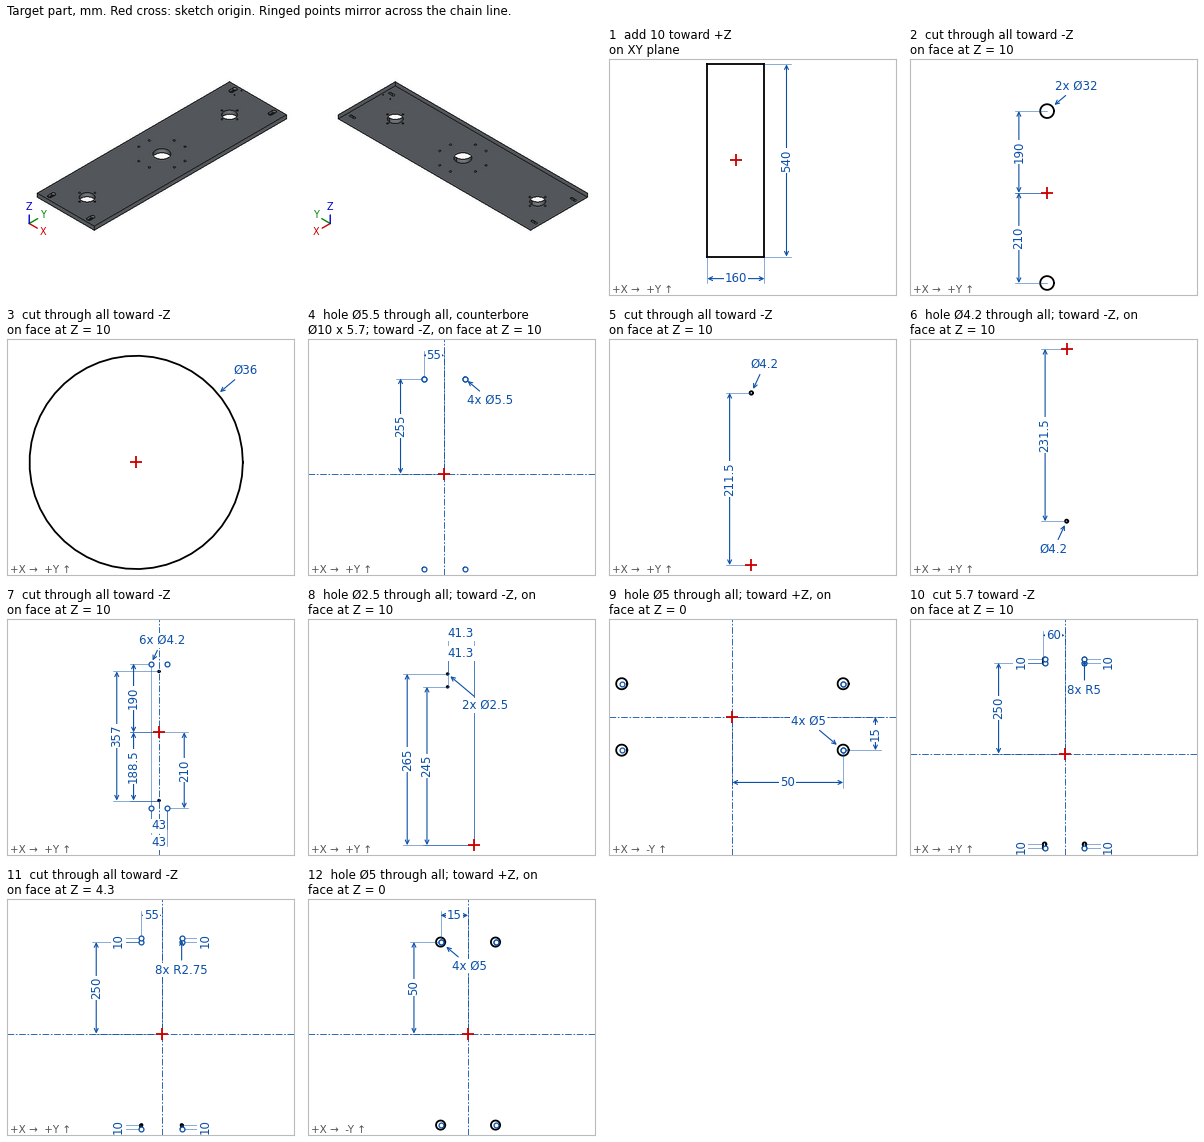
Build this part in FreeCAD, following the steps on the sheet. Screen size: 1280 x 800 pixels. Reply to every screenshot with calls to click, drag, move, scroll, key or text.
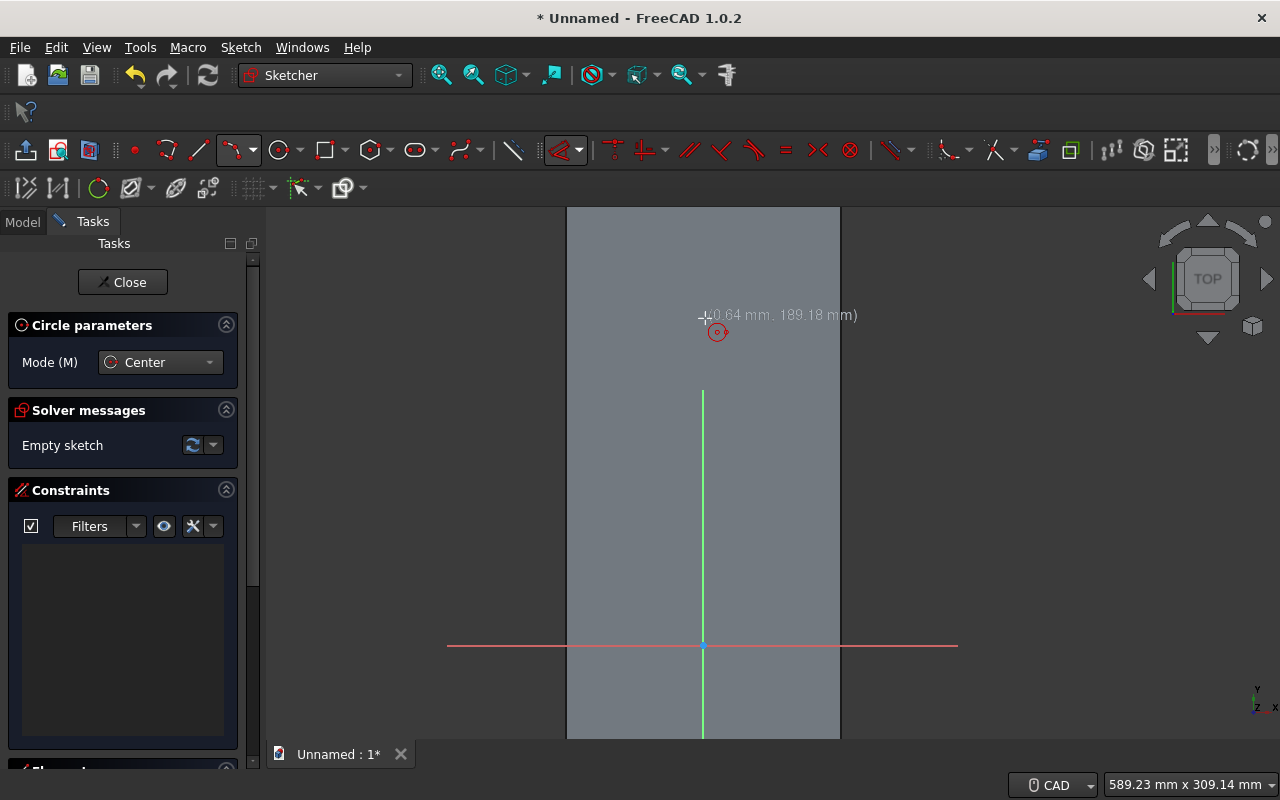
click(703, 319)
move(723, 299)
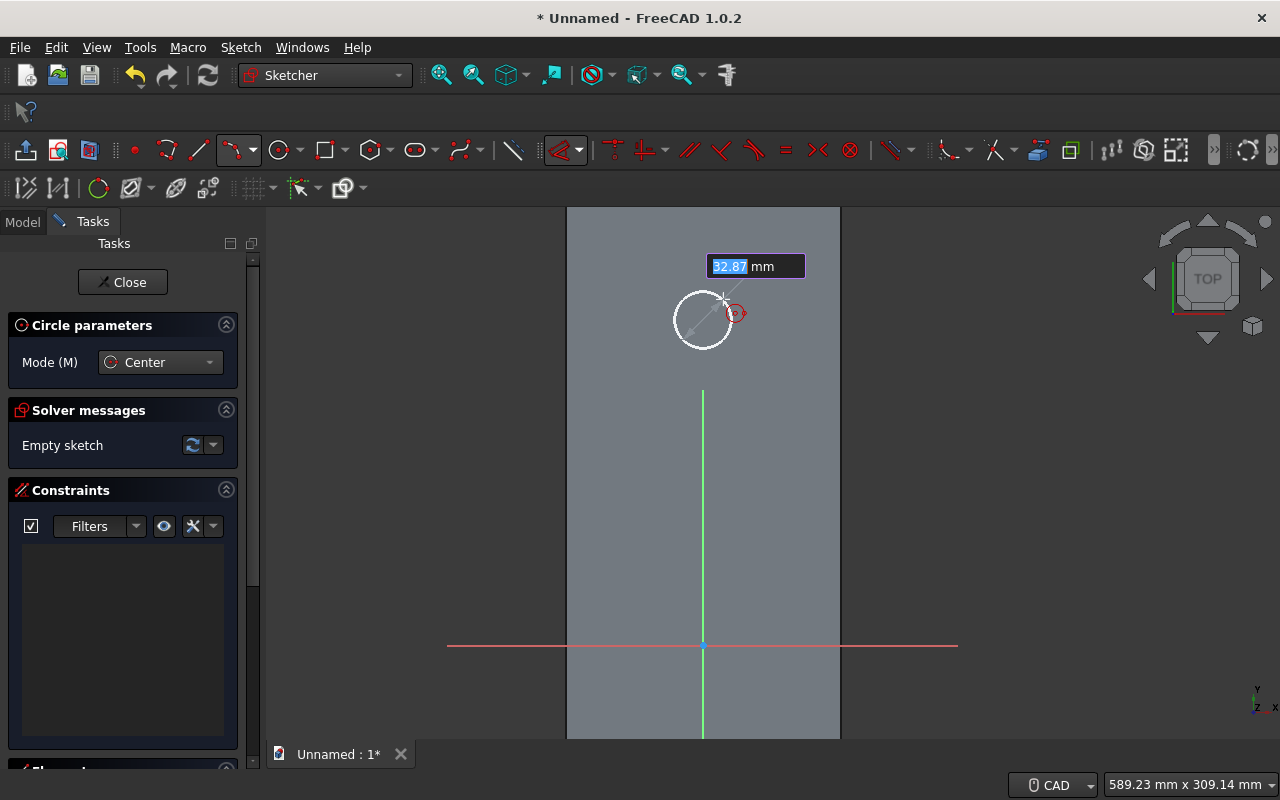
text(32)
key(Return)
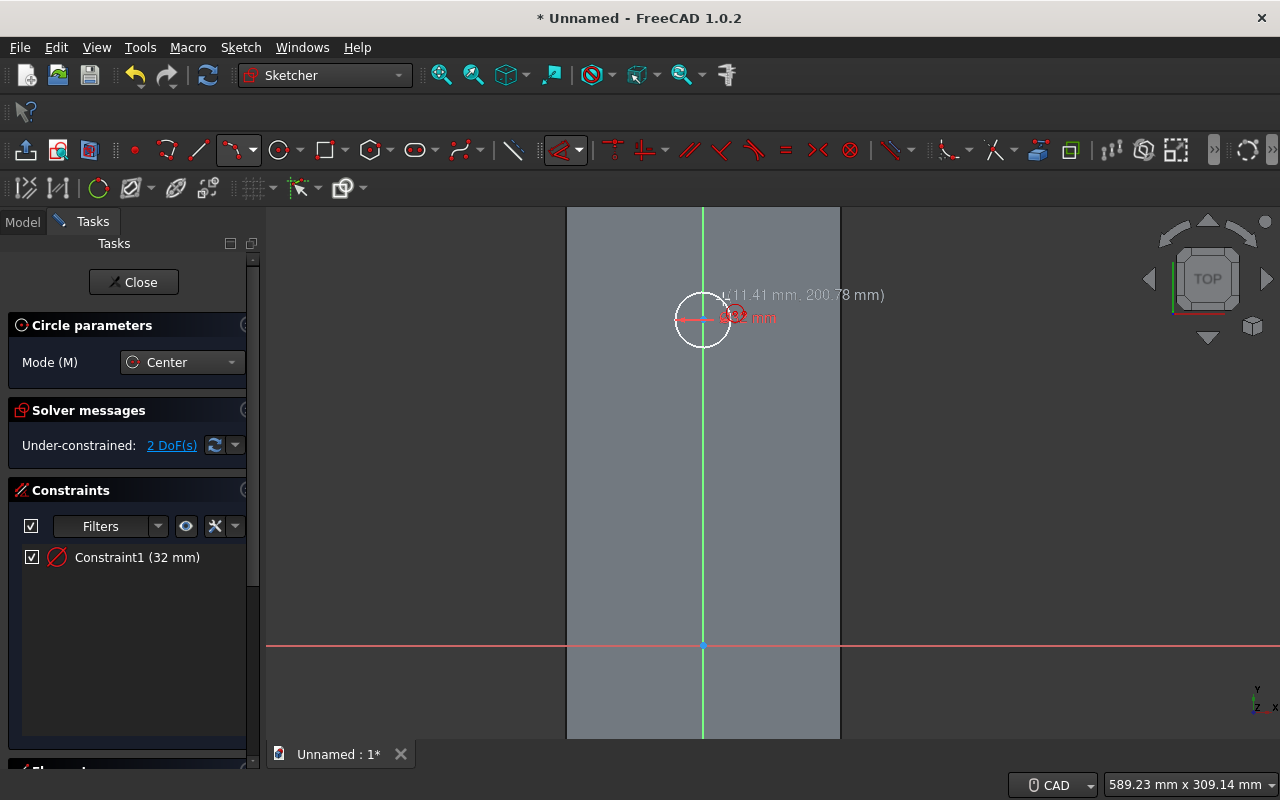
scroll(705, 318, down, 4)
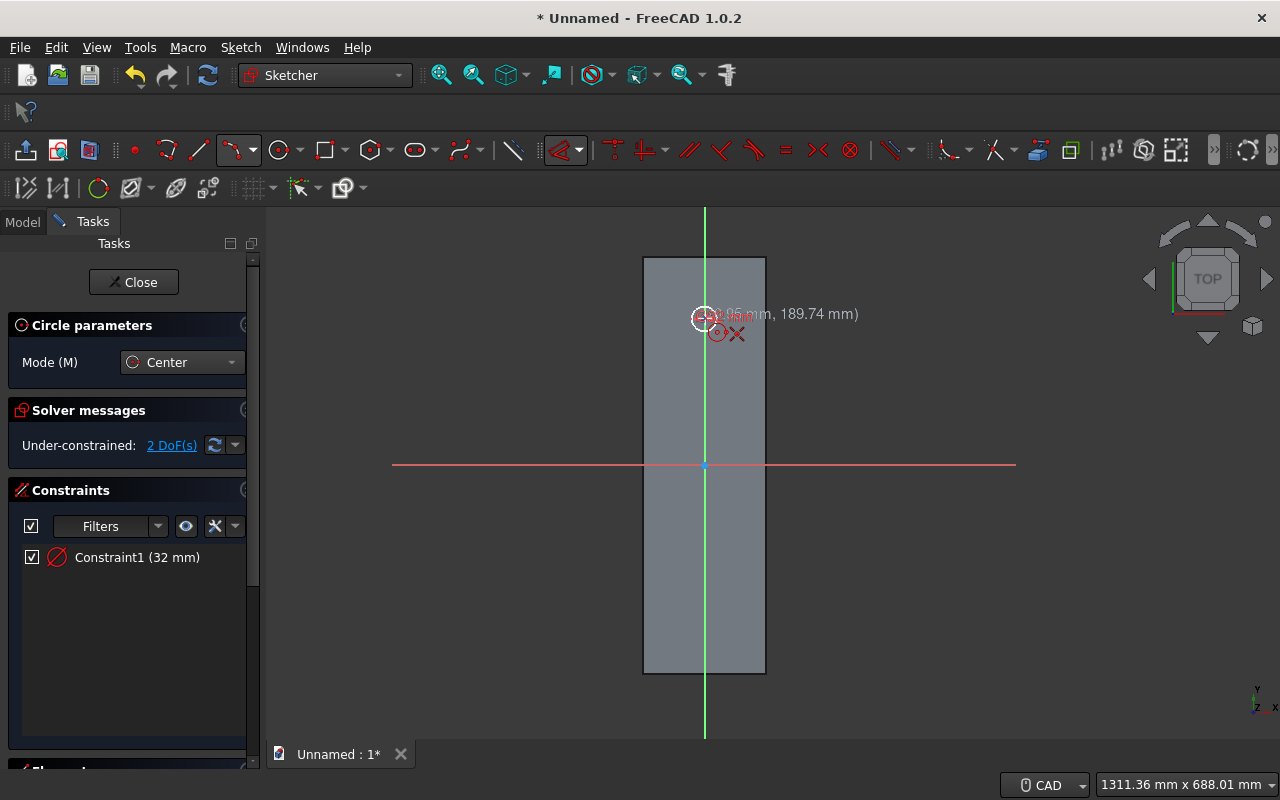
scroll(705, 628, up, 4)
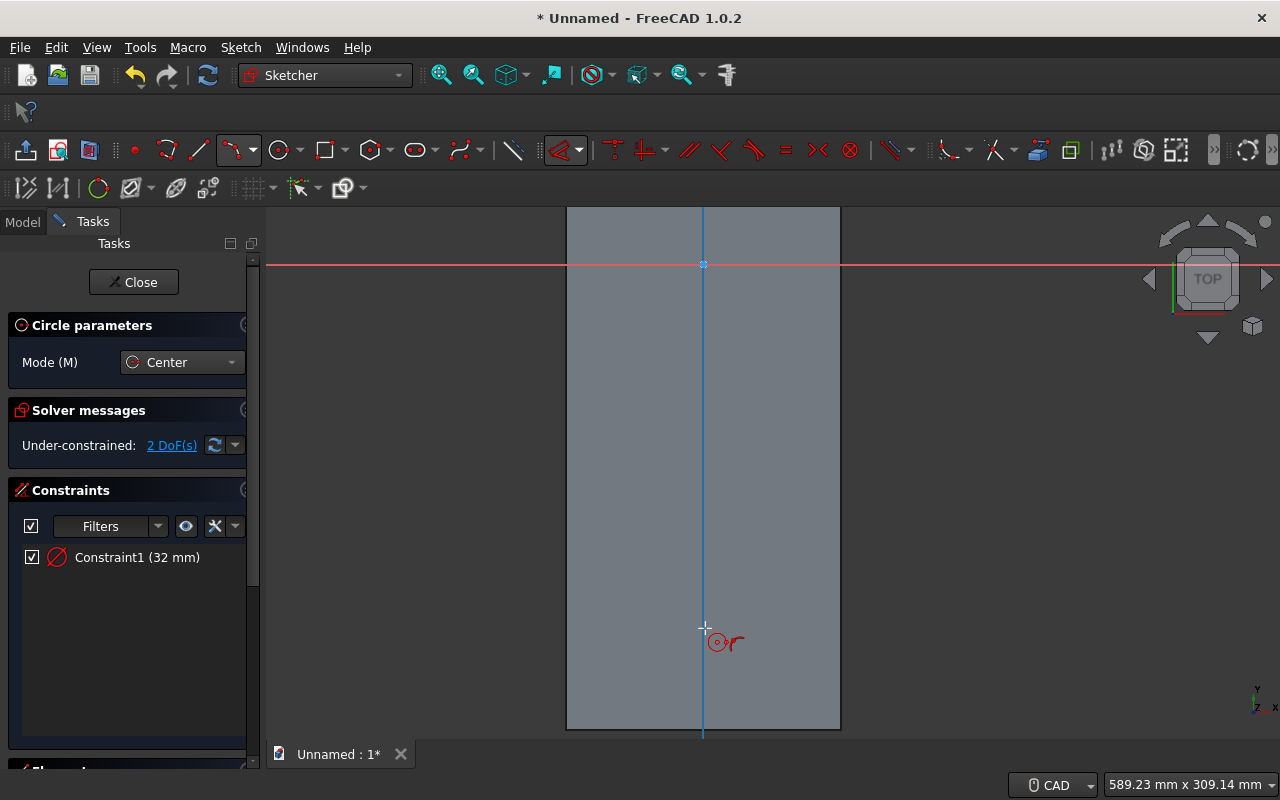
click(703, 626)
move(723, 607)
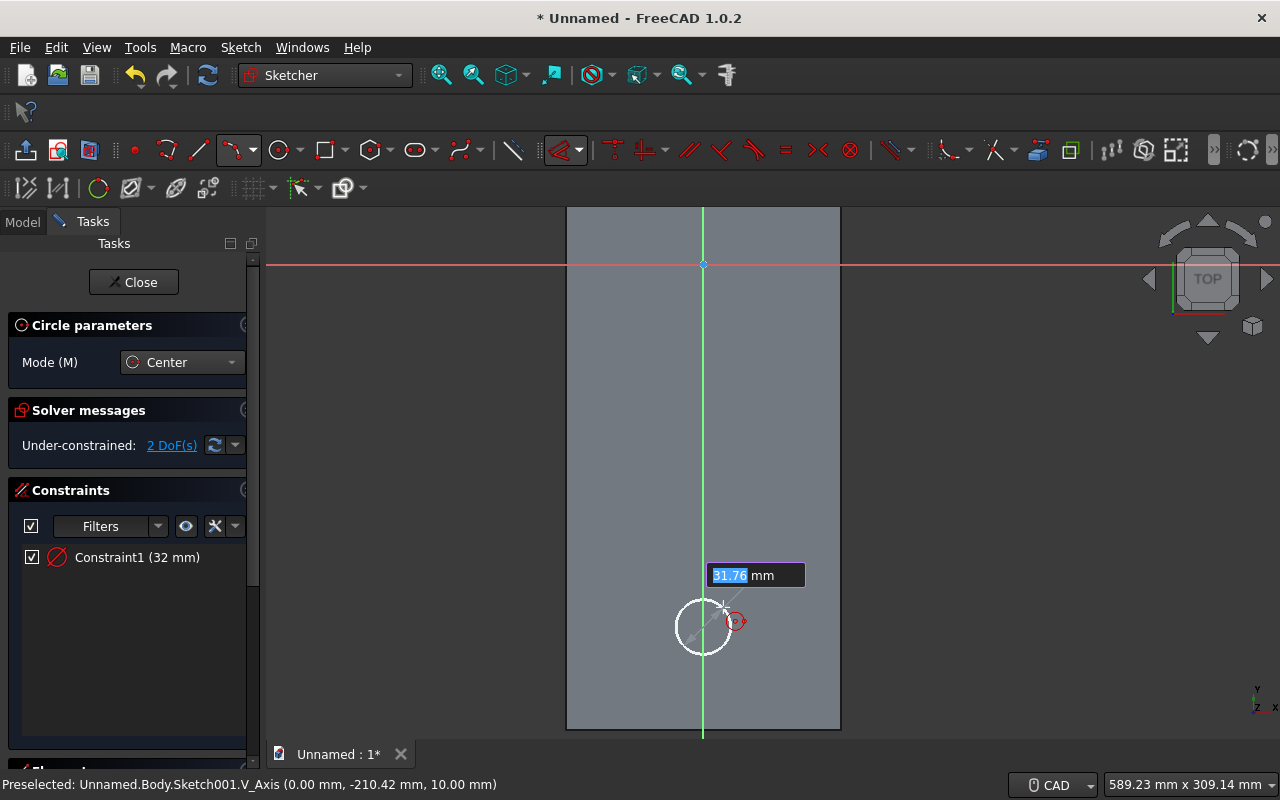
text(32)
key(Return)
key(Escape)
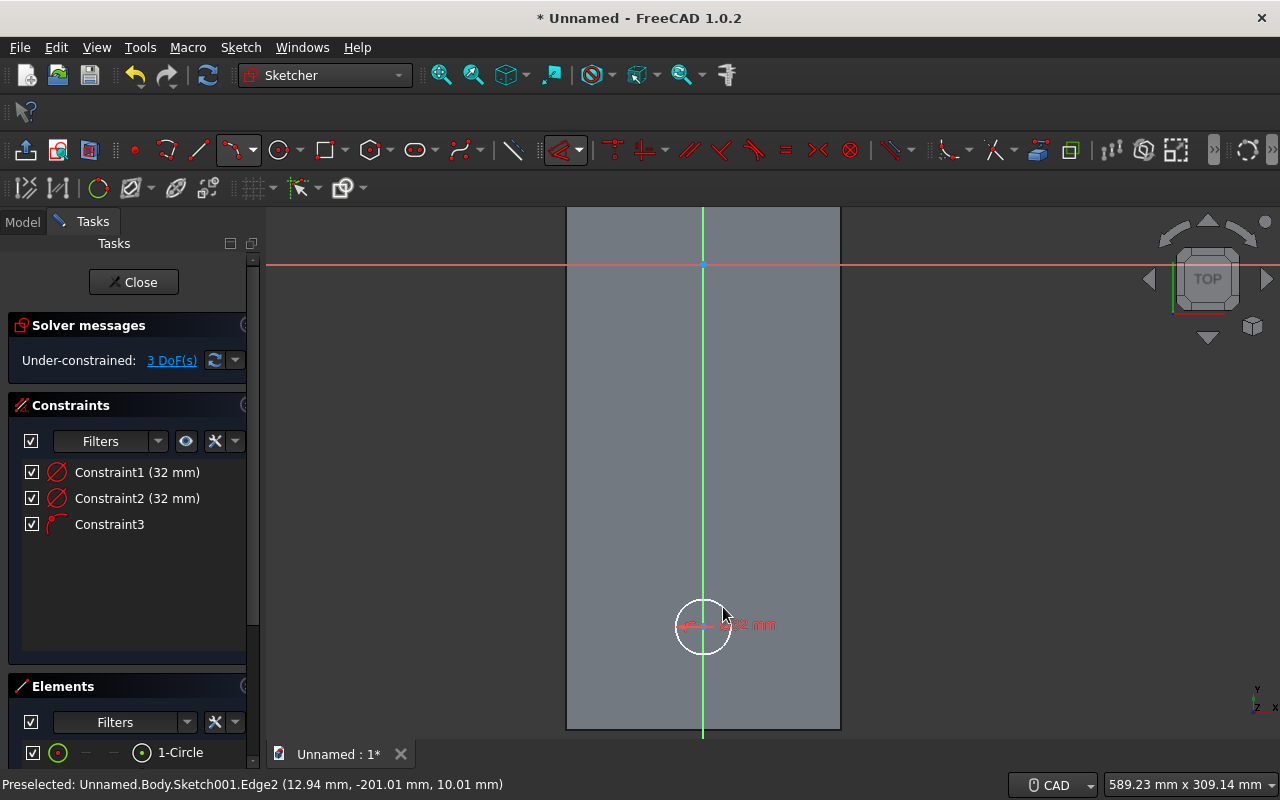
scroll(705, 629, down, 4)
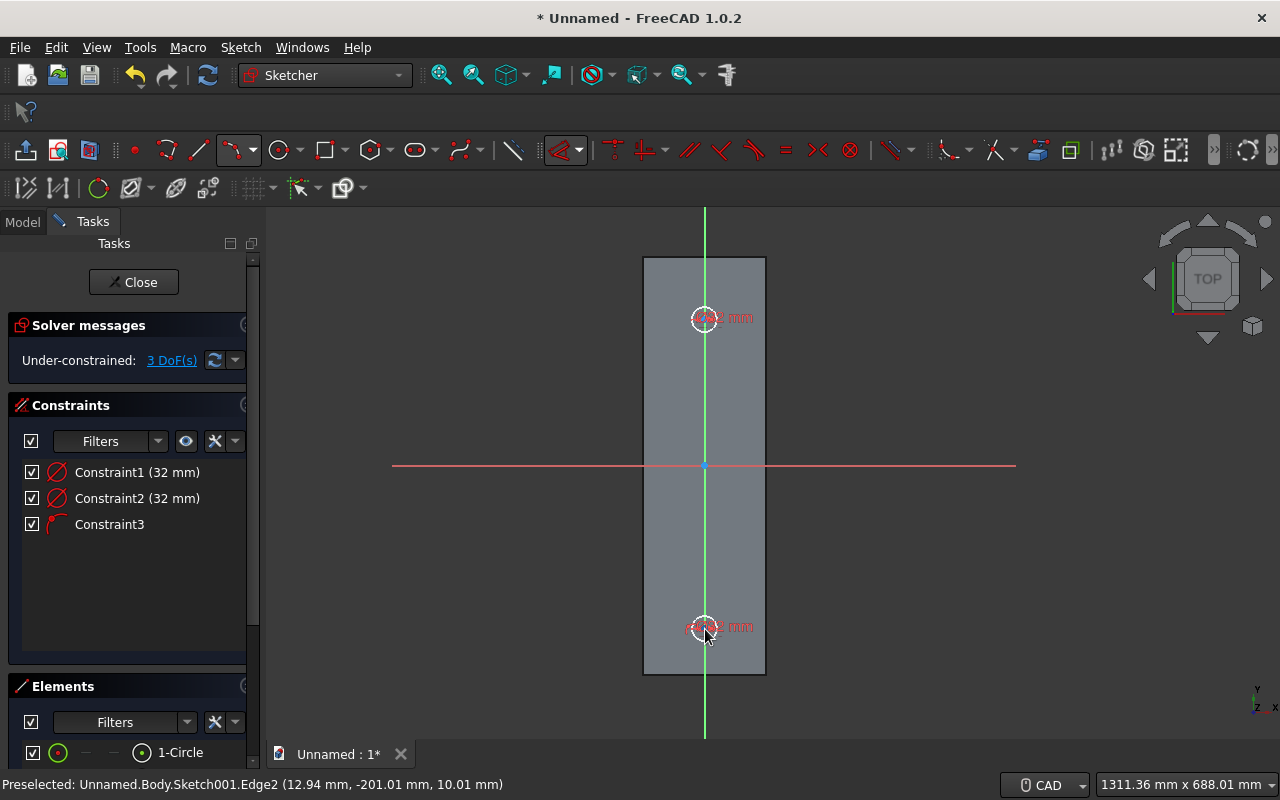
click(704, 320)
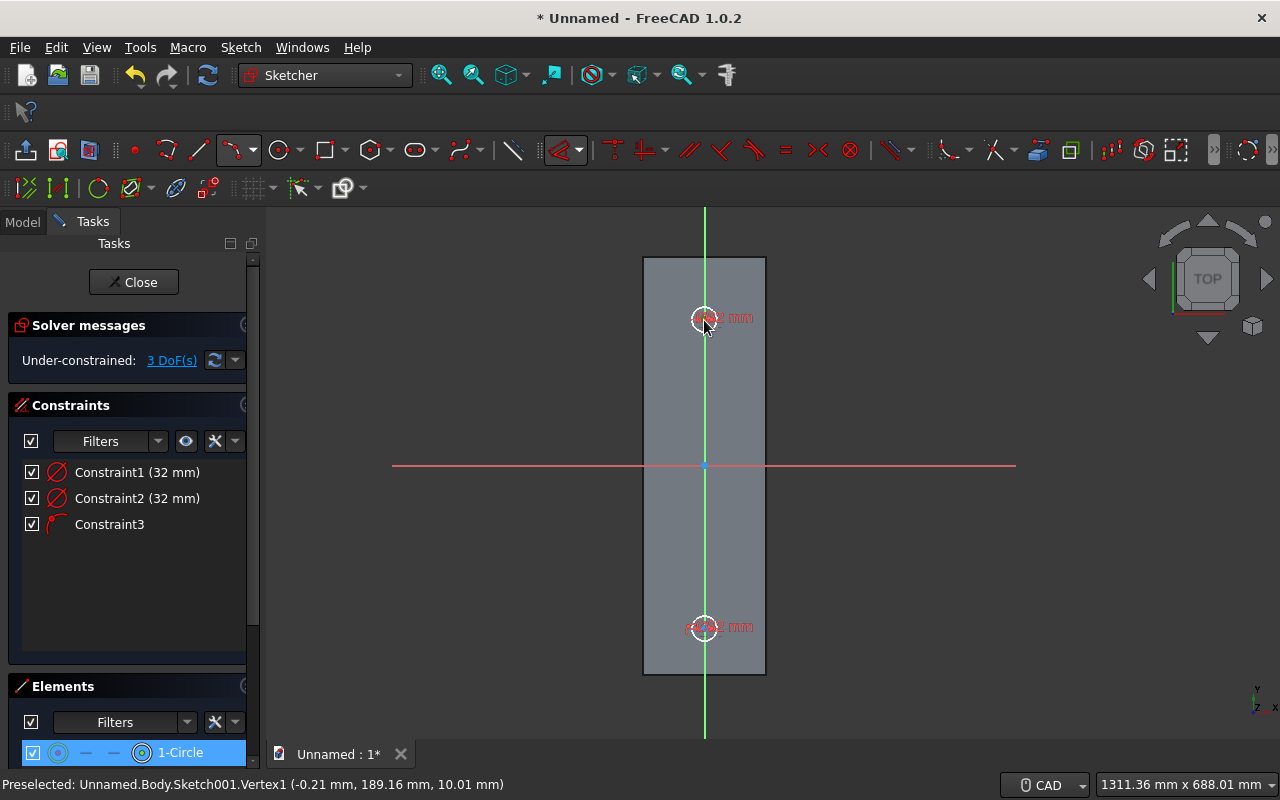
click(705, 677)